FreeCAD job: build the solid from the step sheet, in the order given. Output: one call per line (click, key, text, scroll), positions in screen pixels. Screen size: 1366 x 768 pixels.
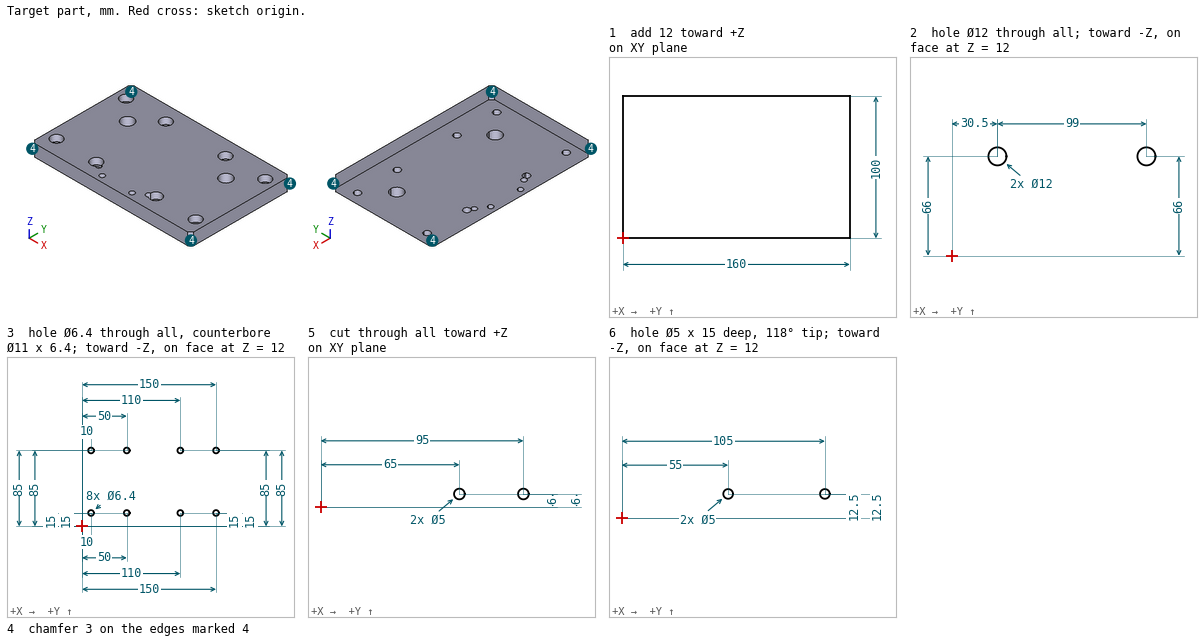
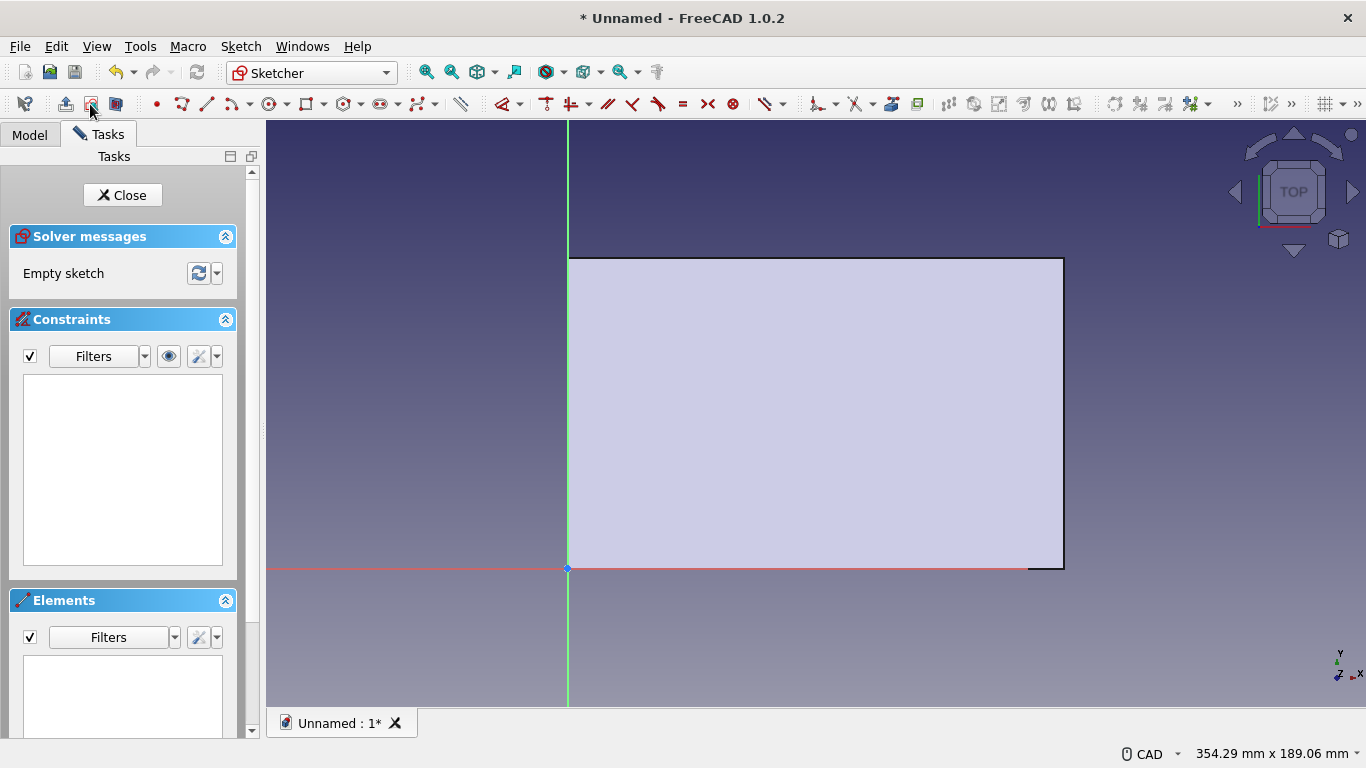
scroll(840, 545, up, 2)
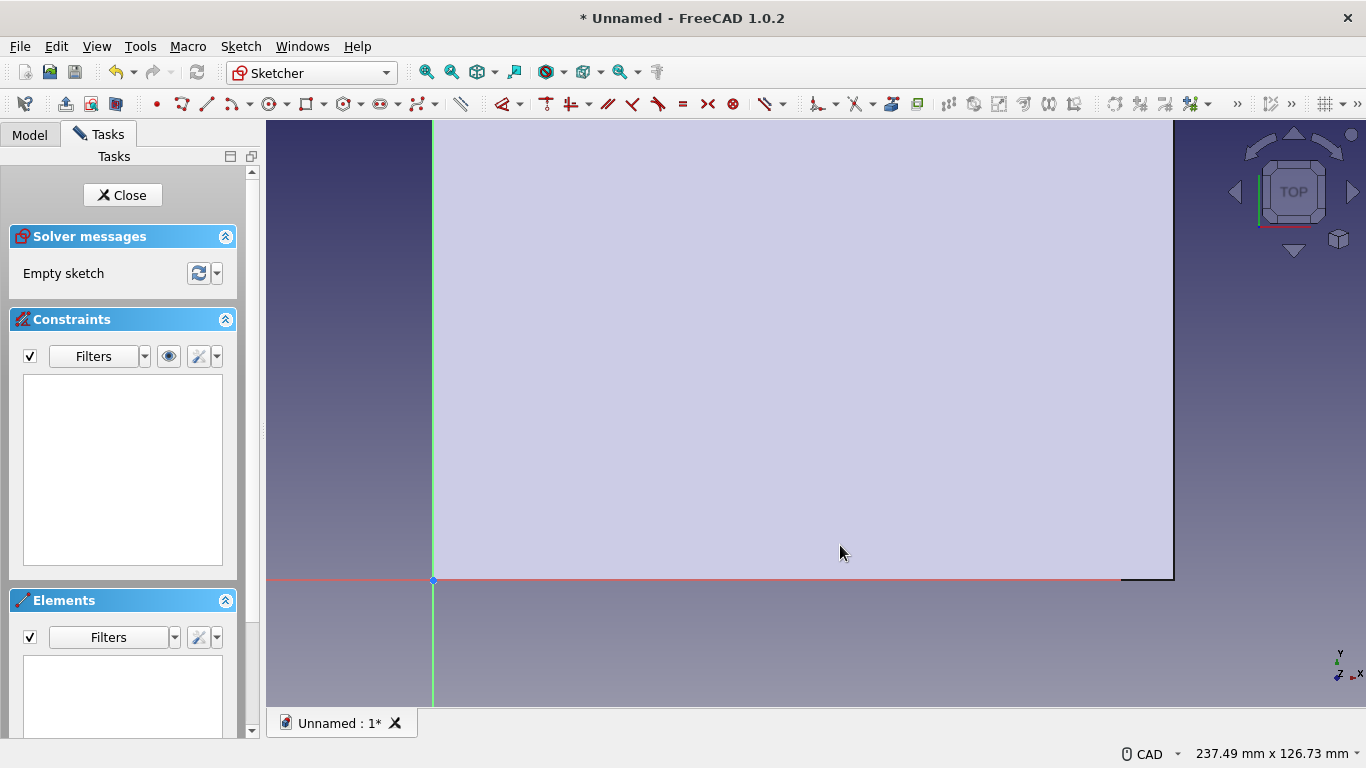
click(268, 104)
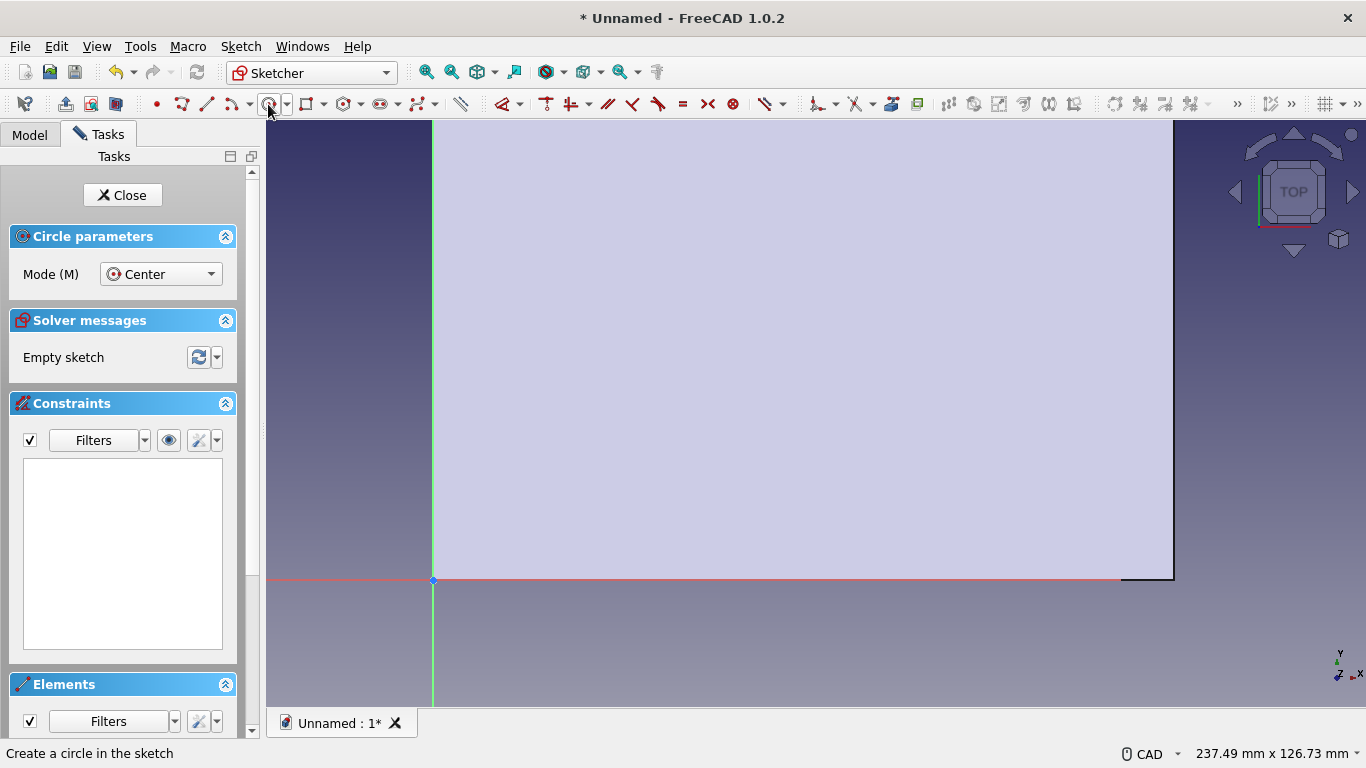
click(575, 274)
click(594, 255)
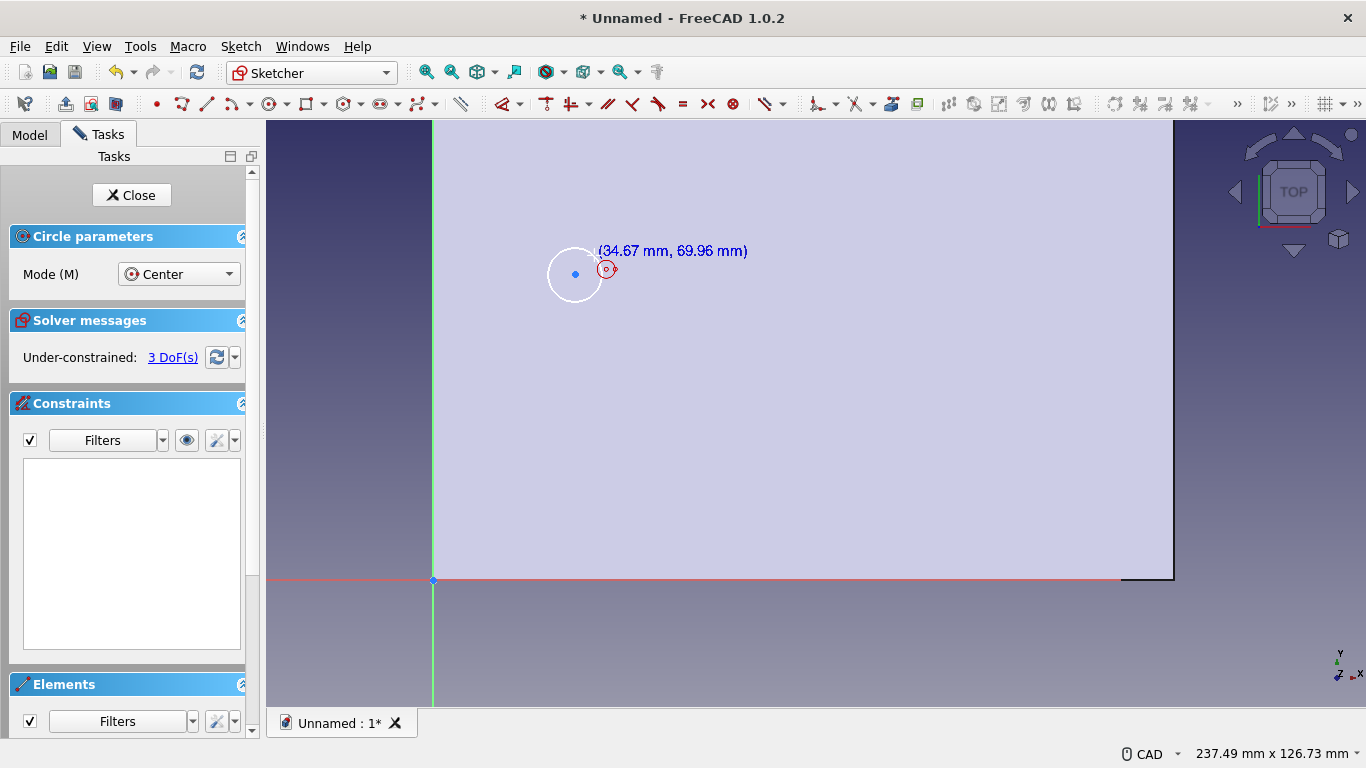
click(1033, 274)
click(1053, 255)
key(Escape)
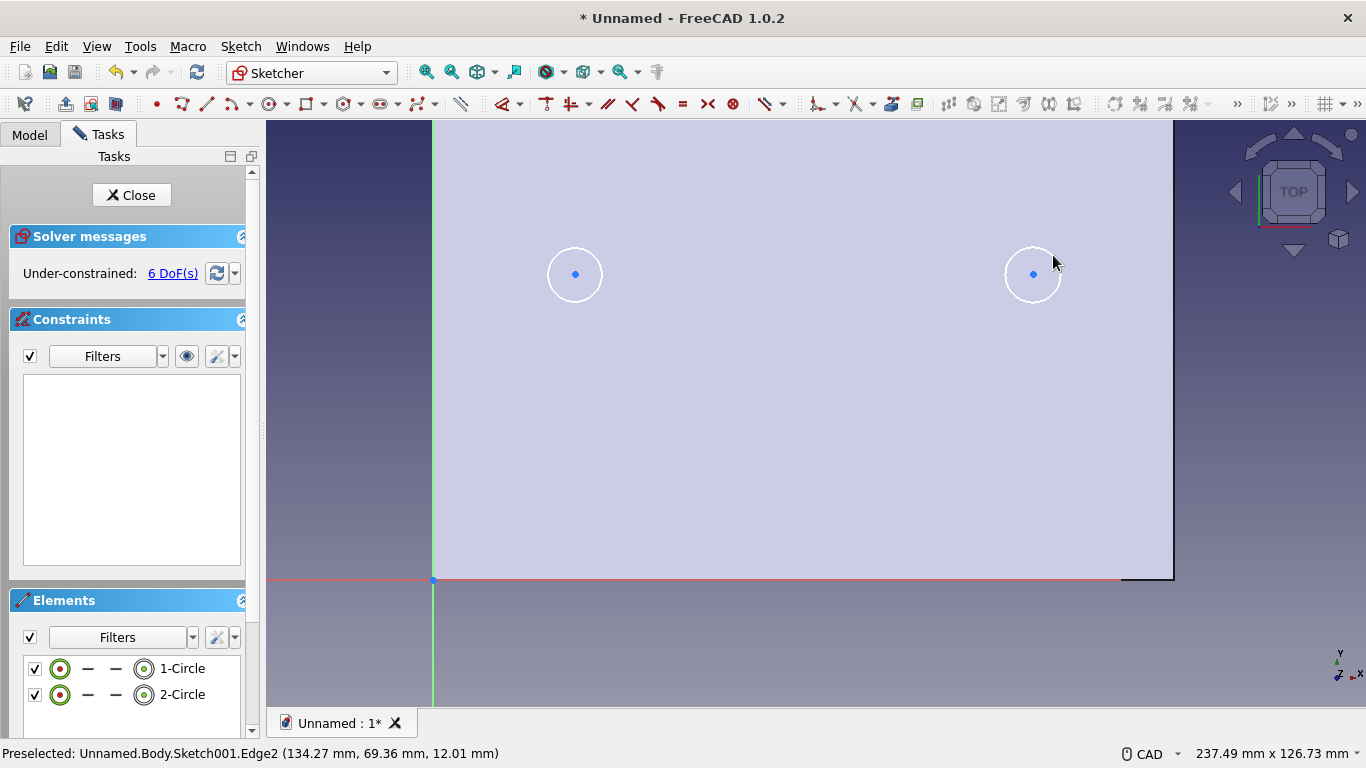
click(594, 256)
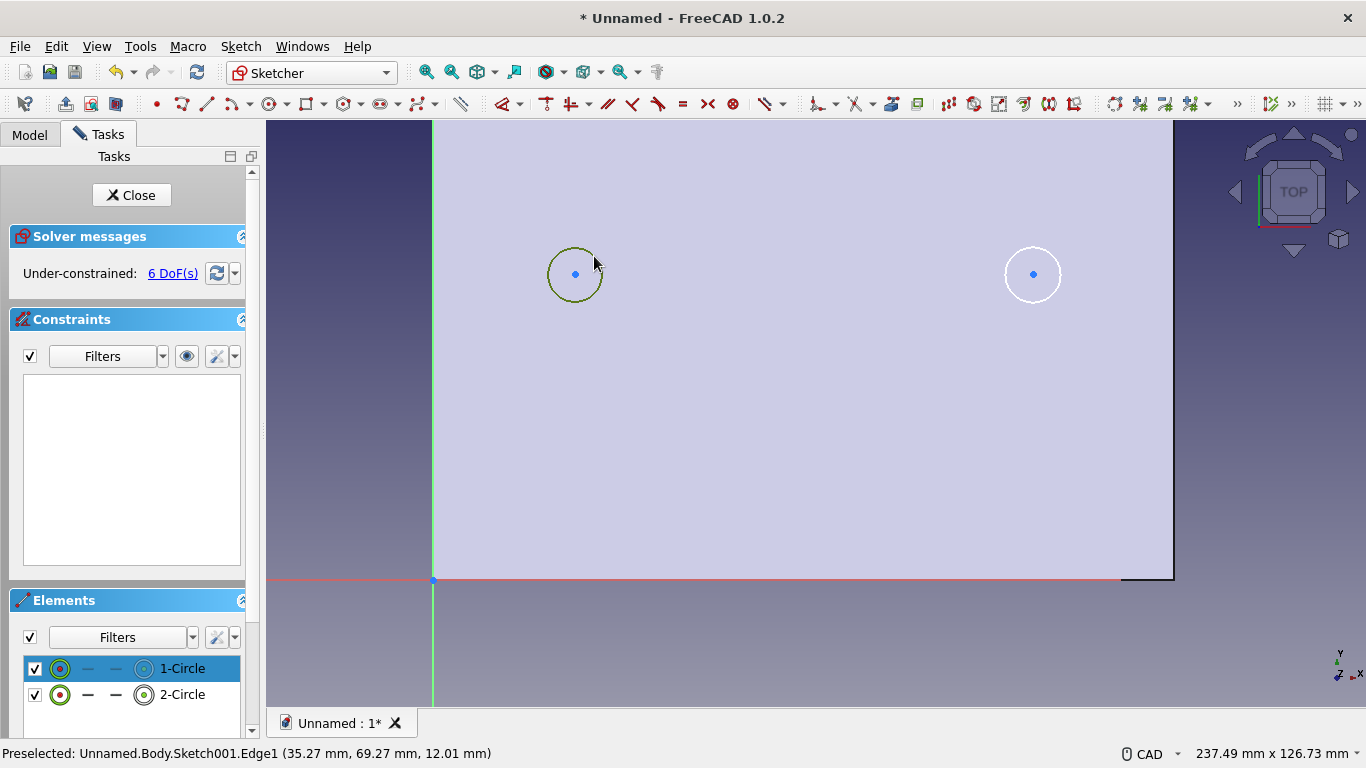
click(1052, 255)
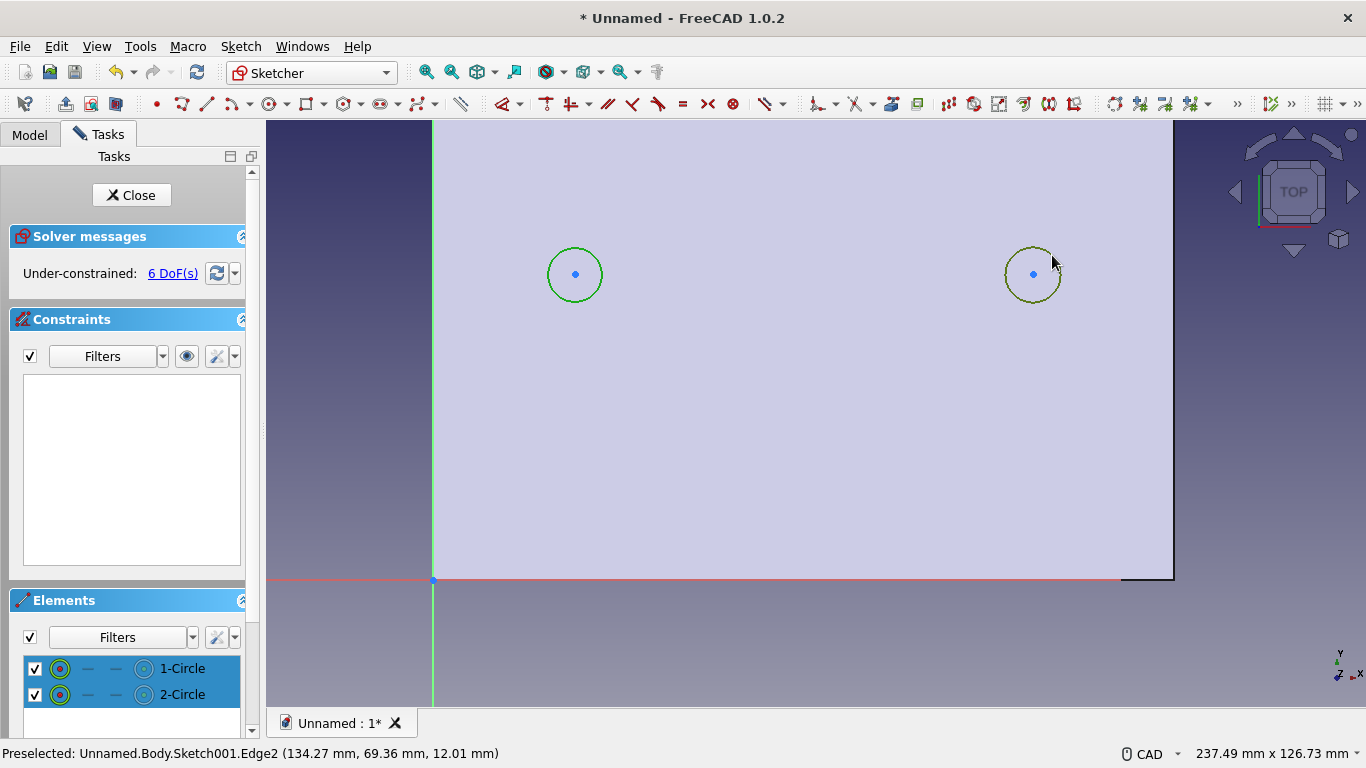
click(683, 104)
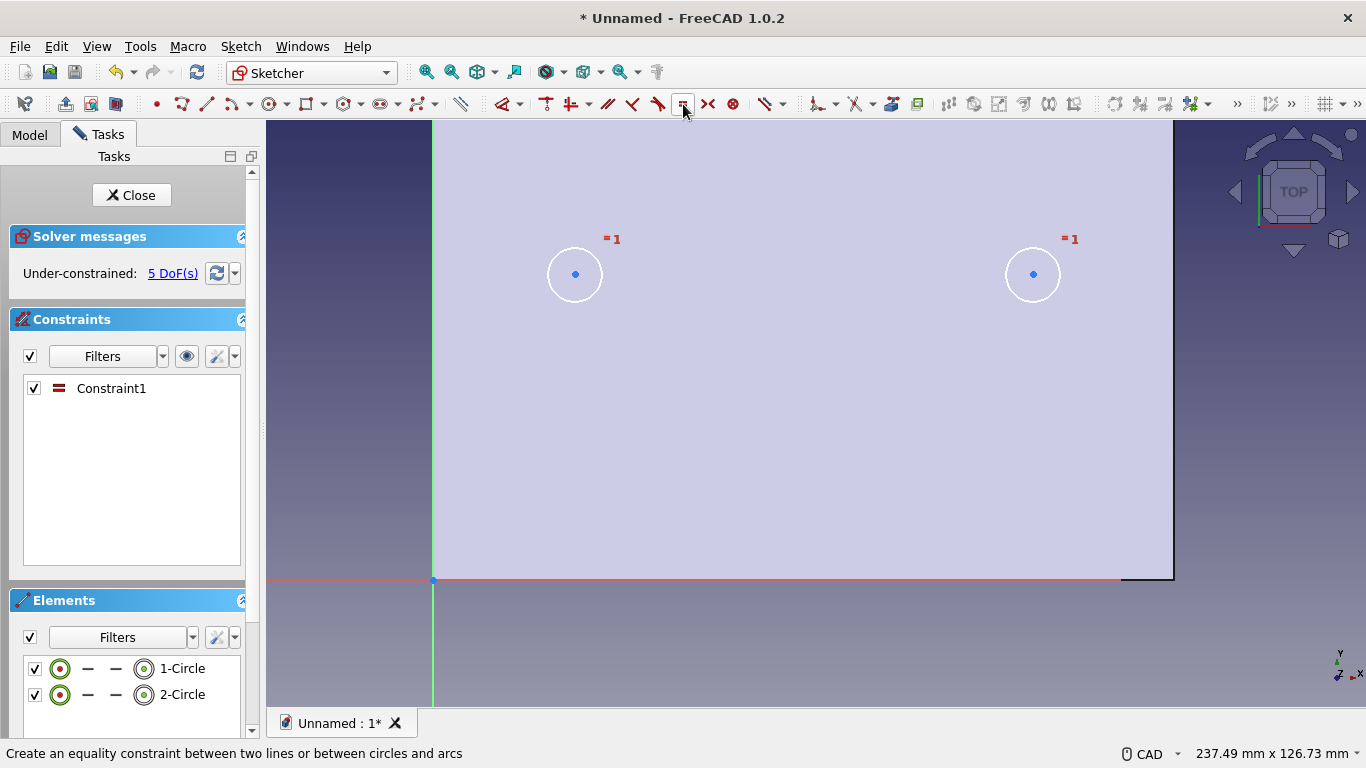
click(594, 256)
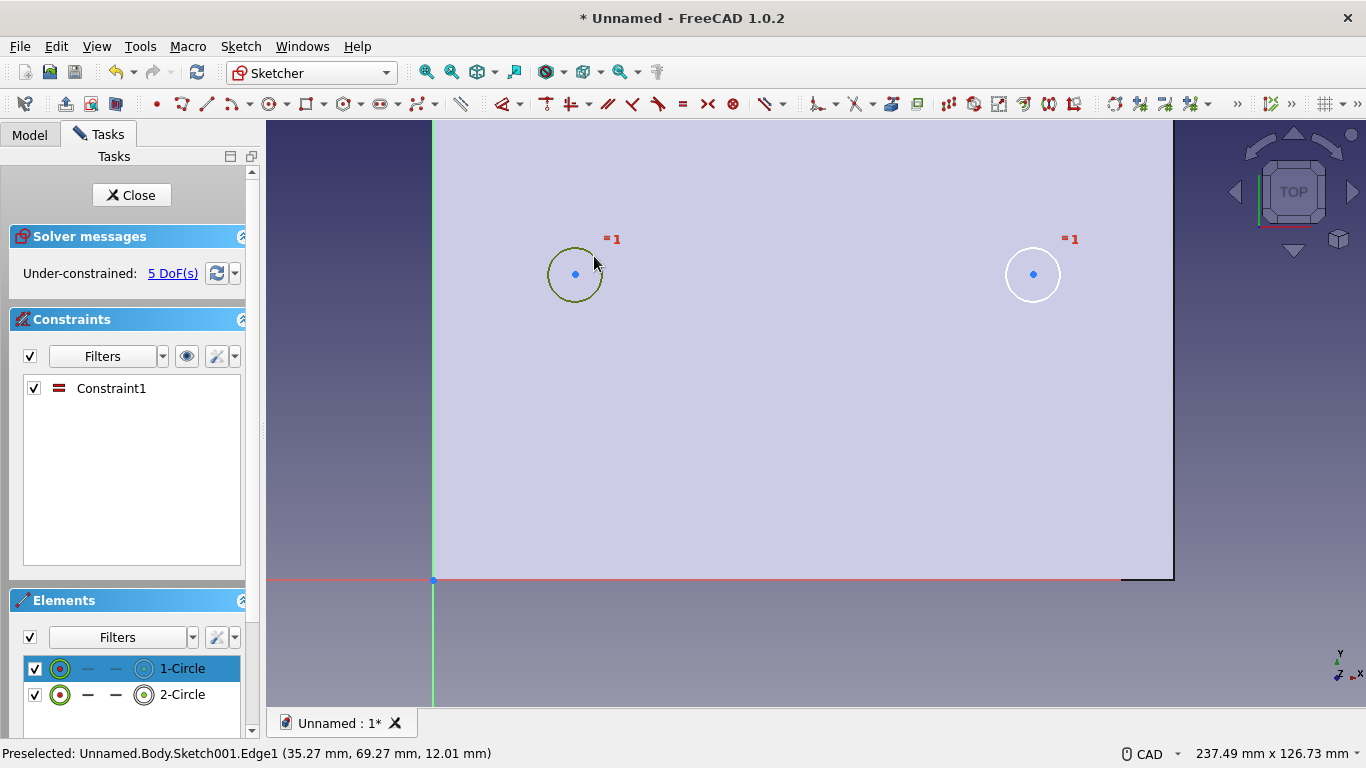
key(k)
key(o)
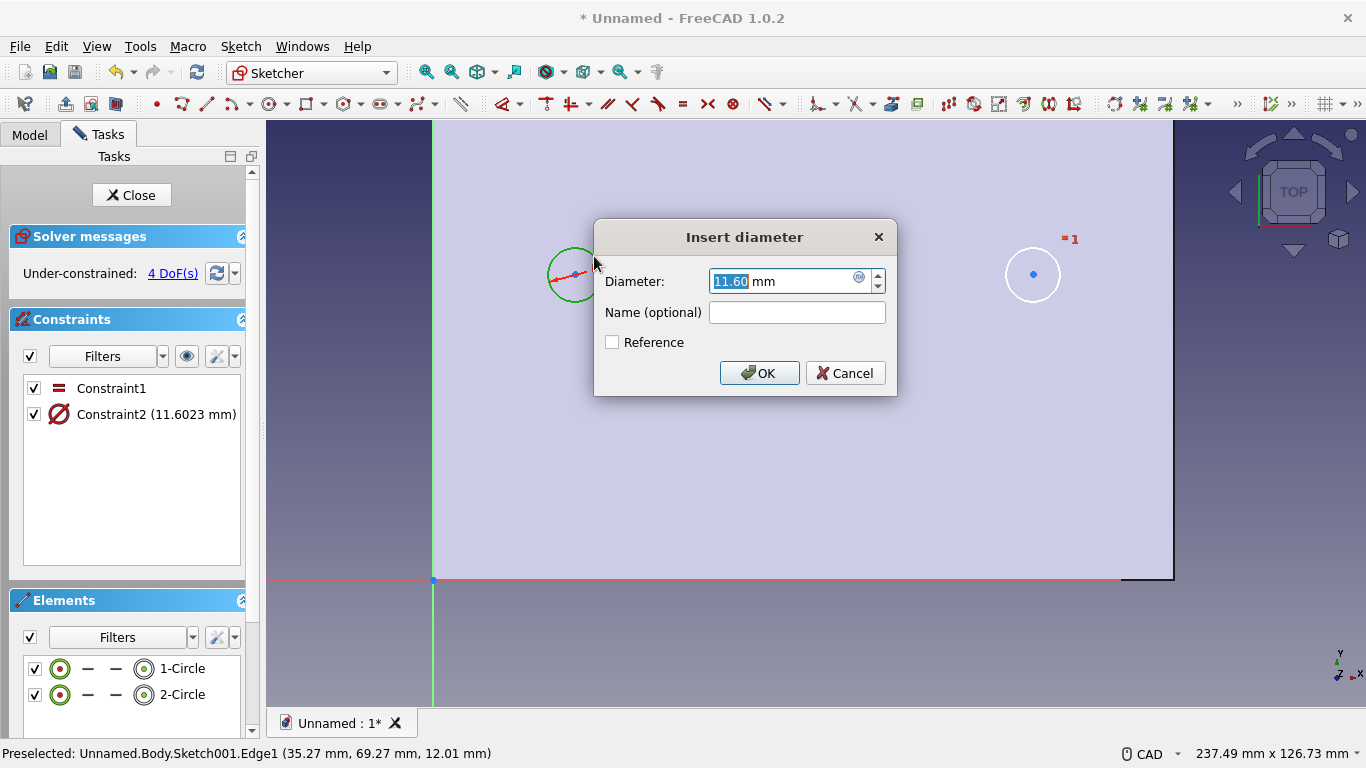
text(12)
key(Return)